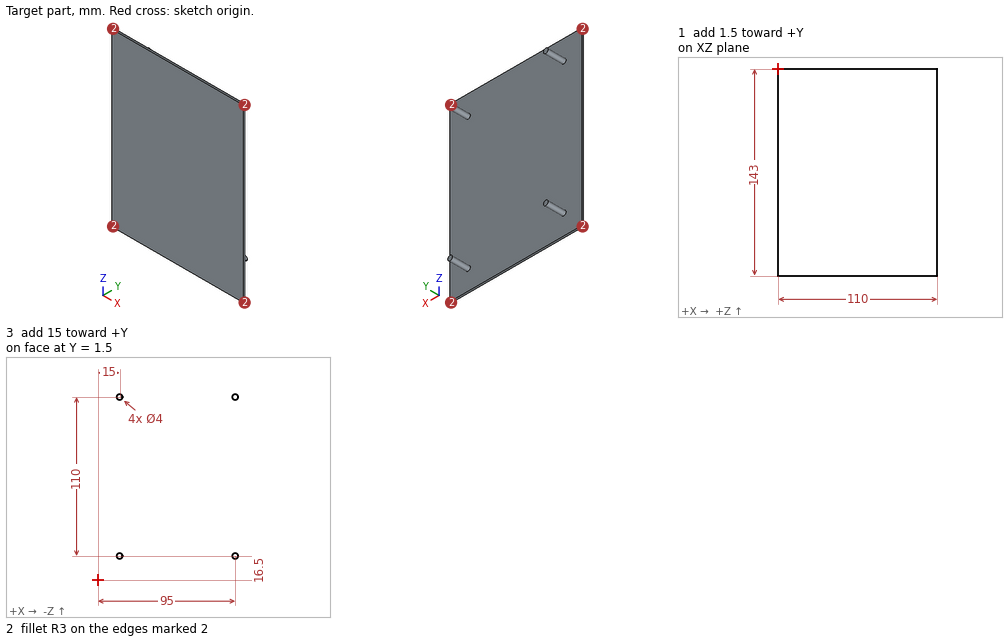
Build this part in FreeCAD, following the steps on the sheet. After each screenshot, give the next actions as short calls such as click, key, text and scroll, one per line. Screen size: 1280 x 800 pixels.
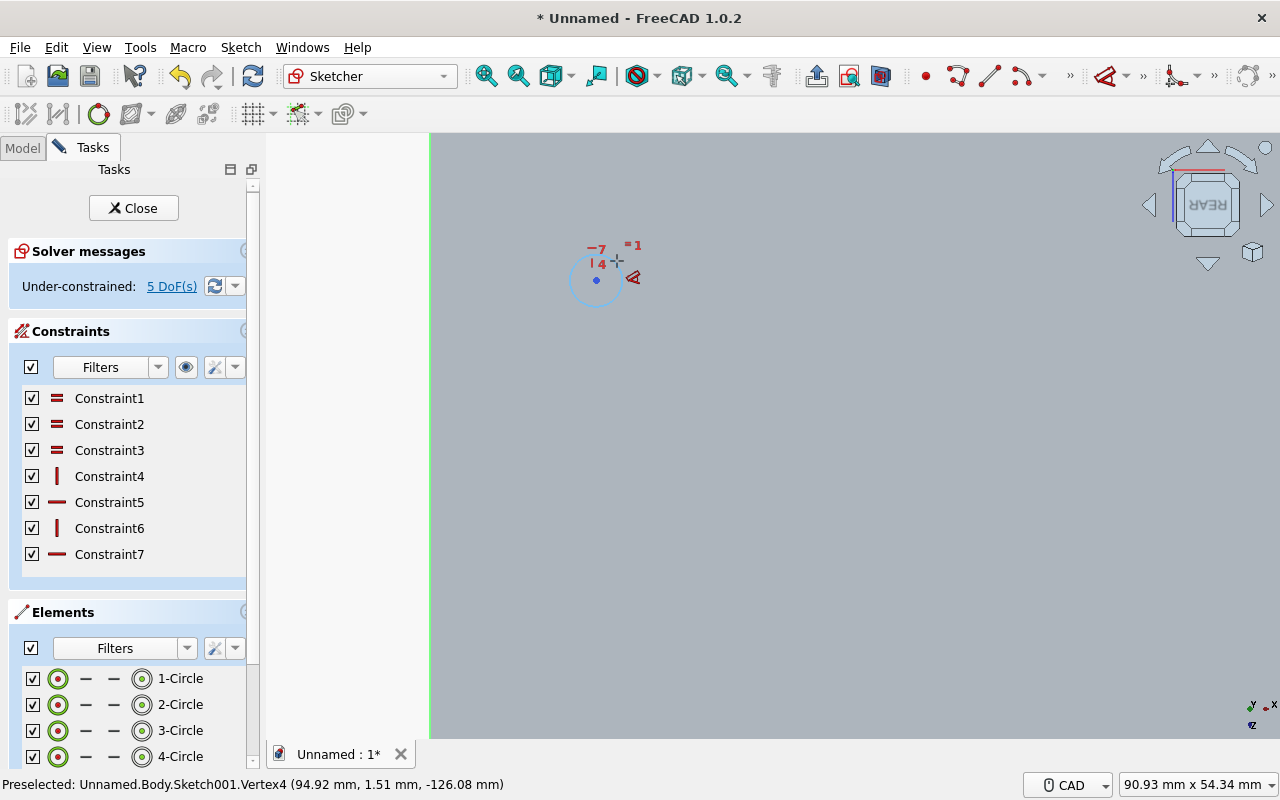
click(614, 262)
click(636, 239)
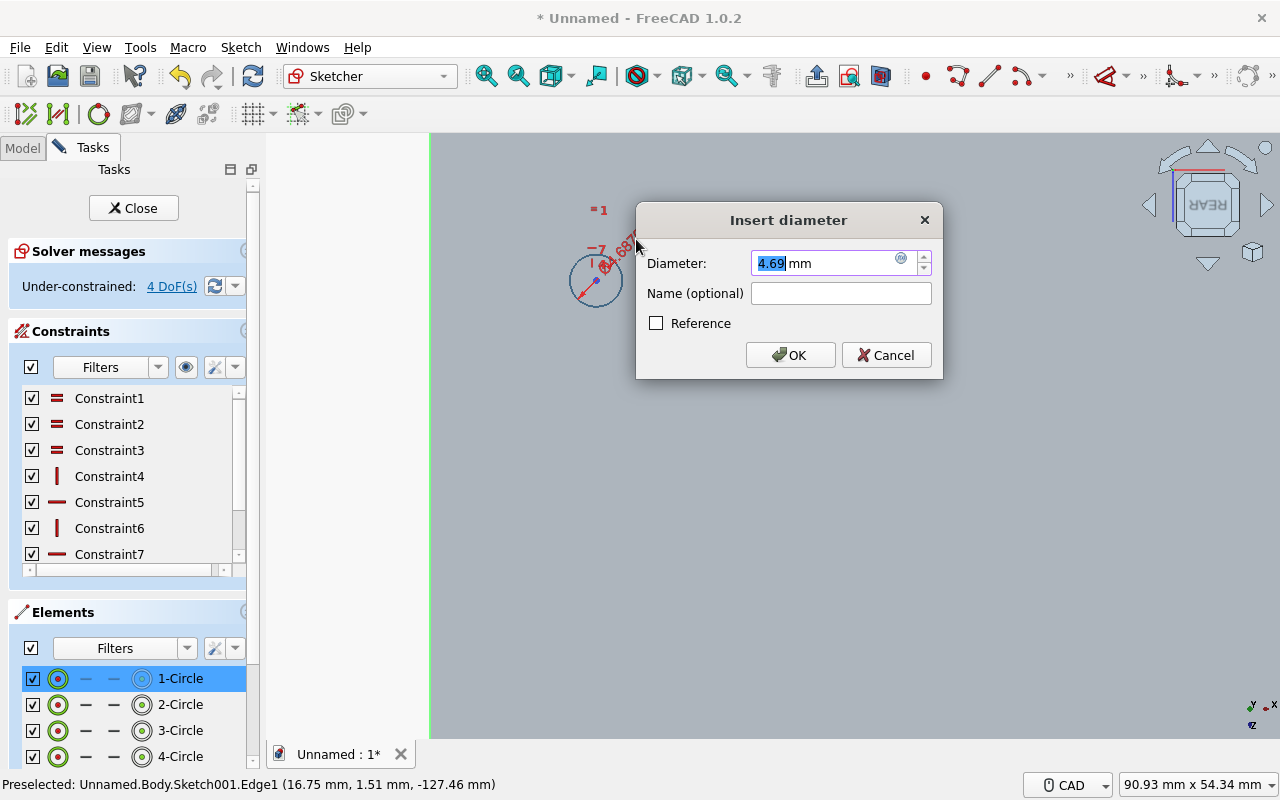
text(4)
key(Return)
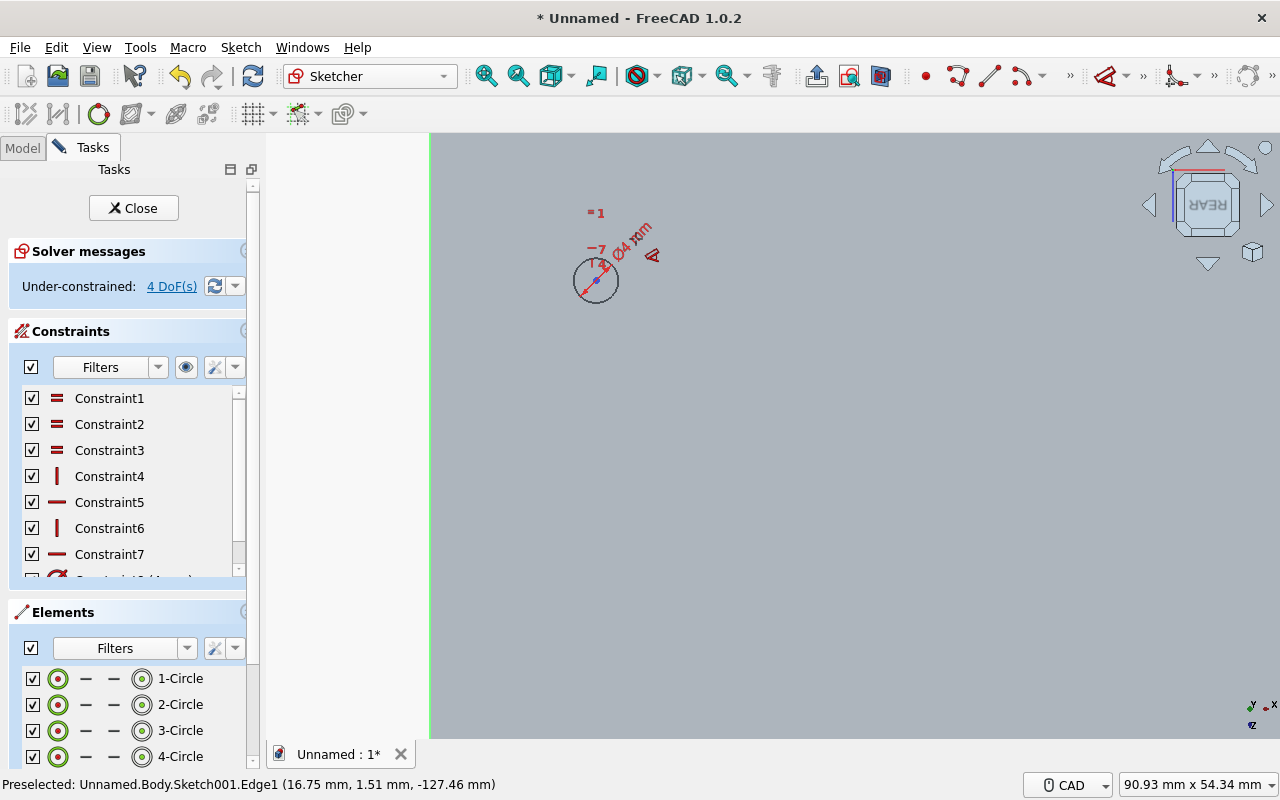
click(596, 281)
click(513, 247)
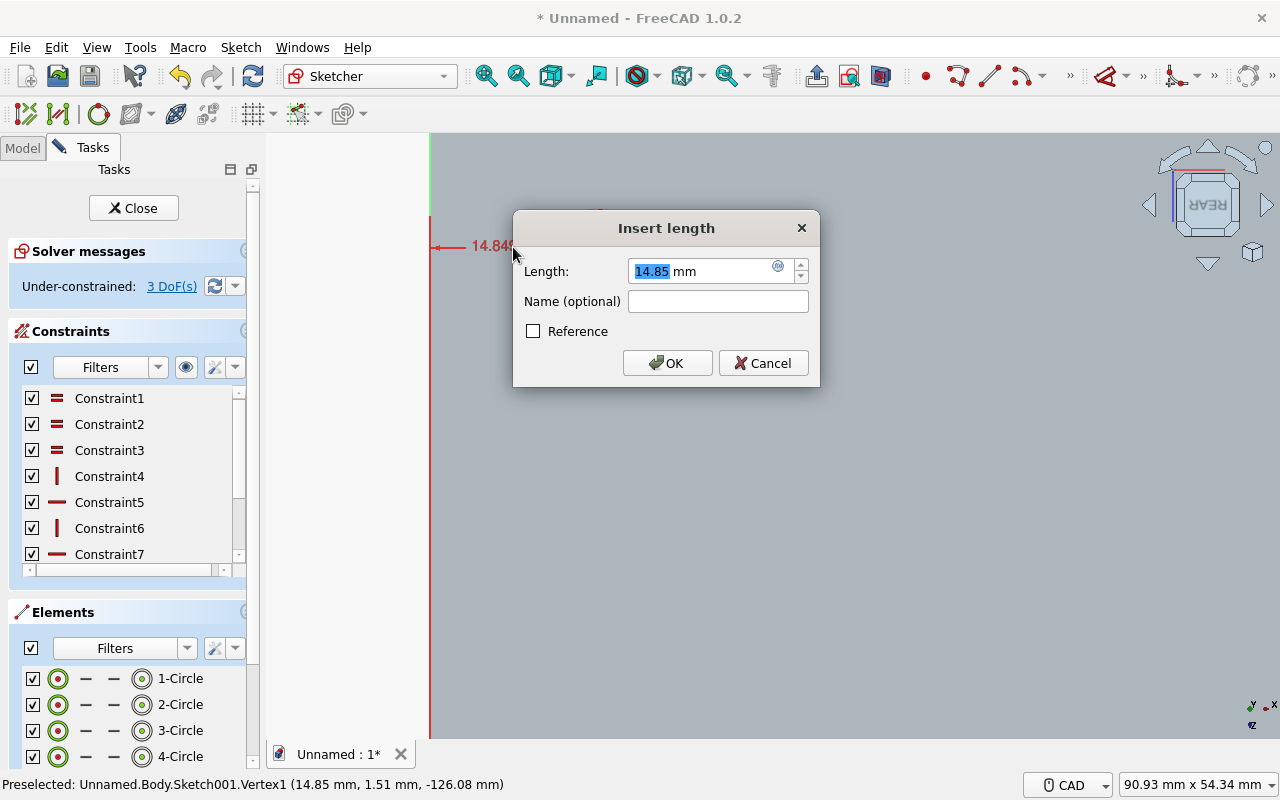
text(15)
key(Return)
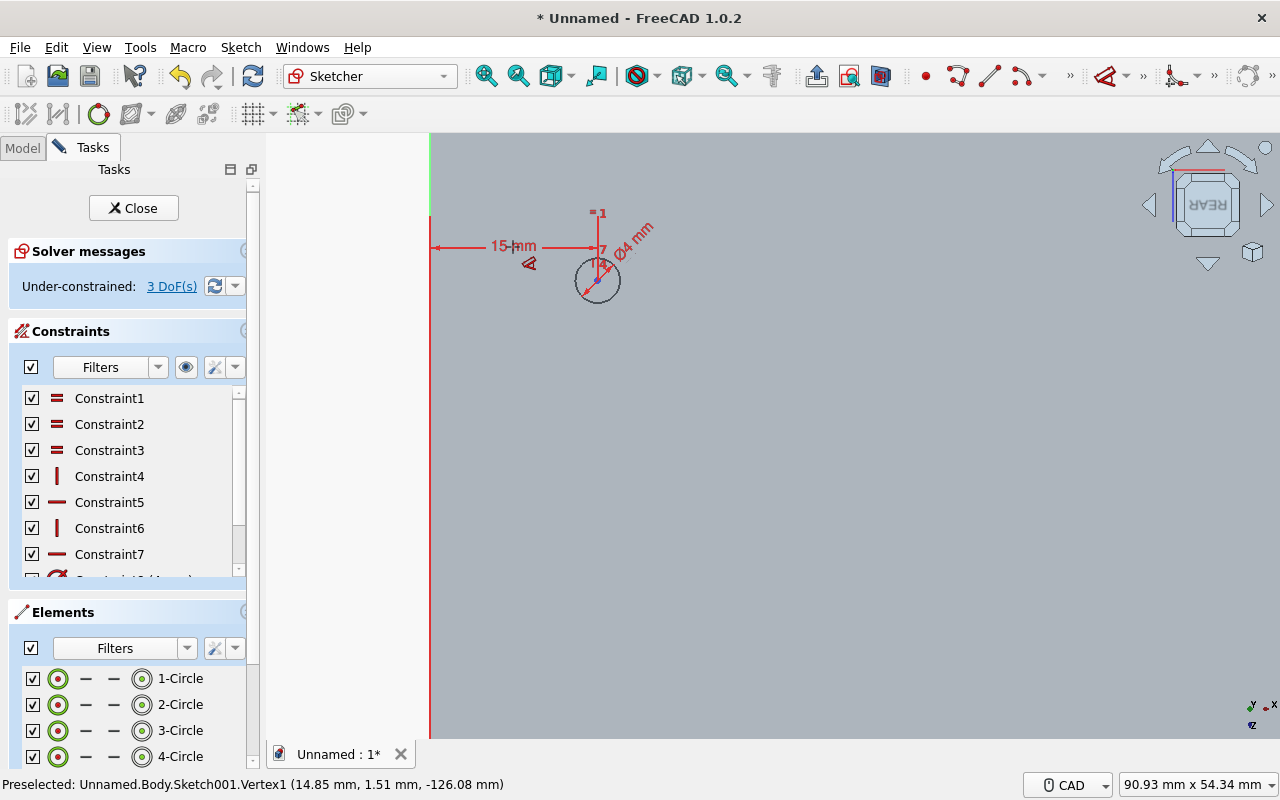
scroll(617, 261, down, 7)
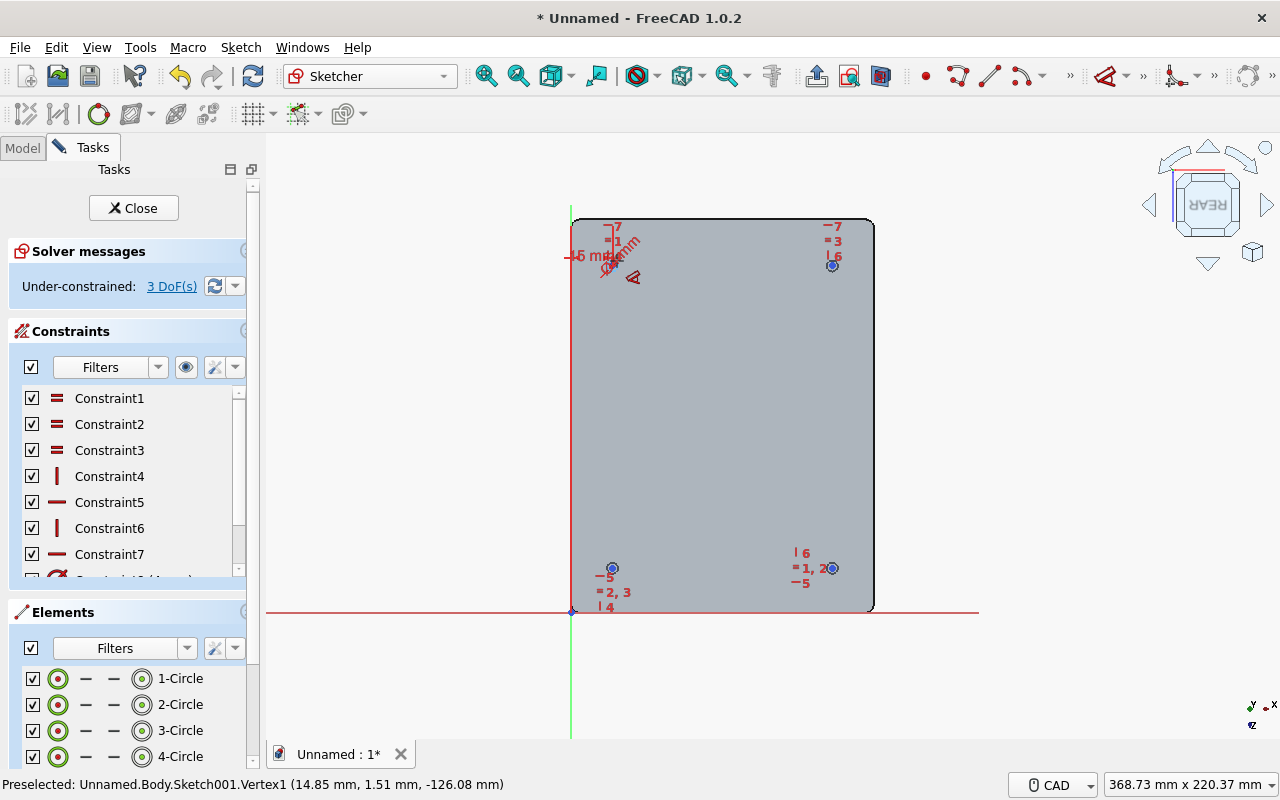
click(832, 568)
click(702, 647)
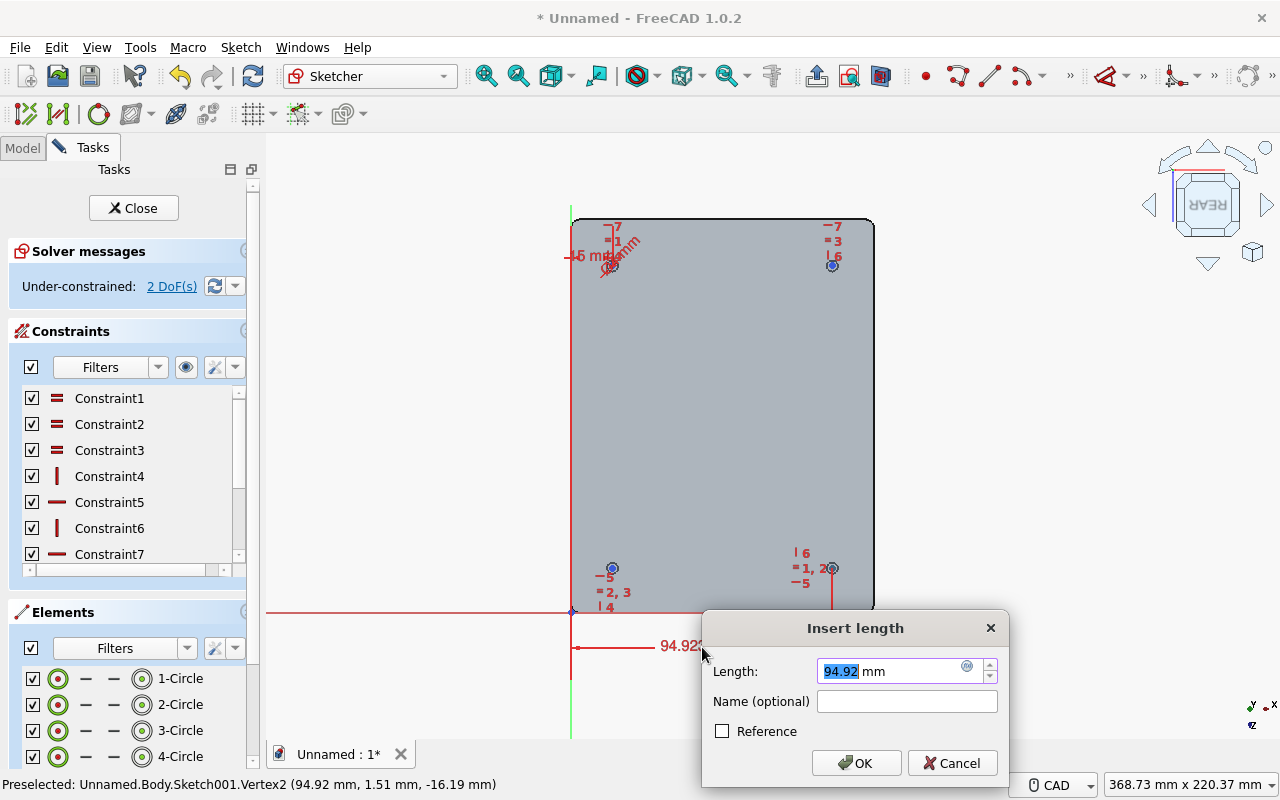
text(95)
key(Return)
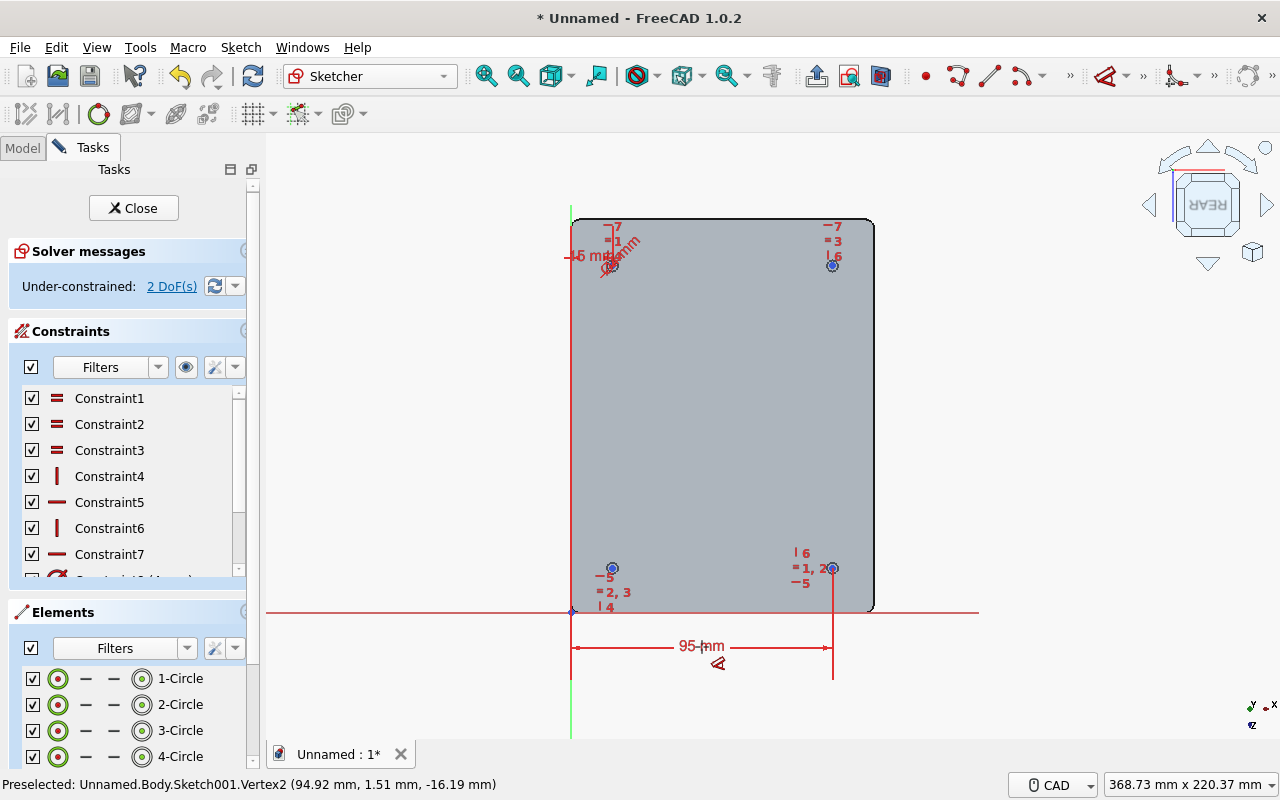
click(833, 568)
click(537, 590)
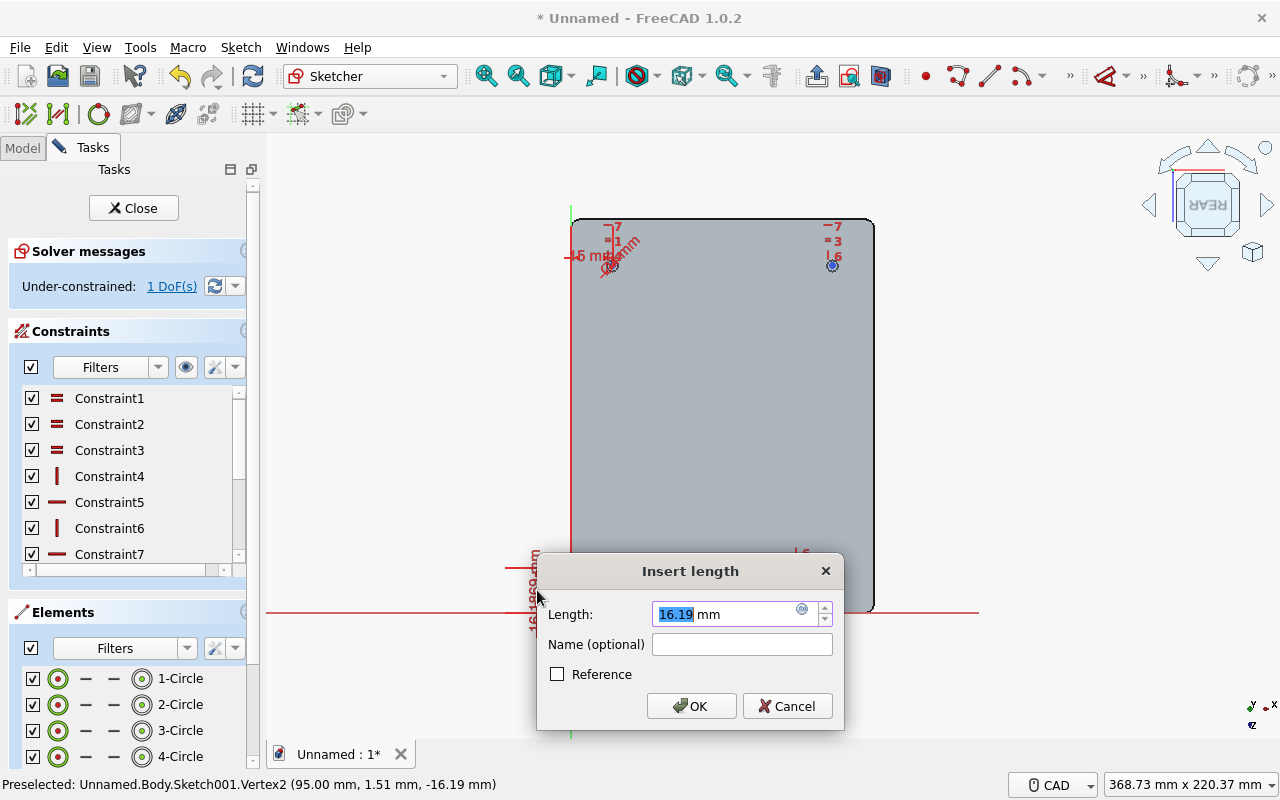
text(16.5)
key(Return)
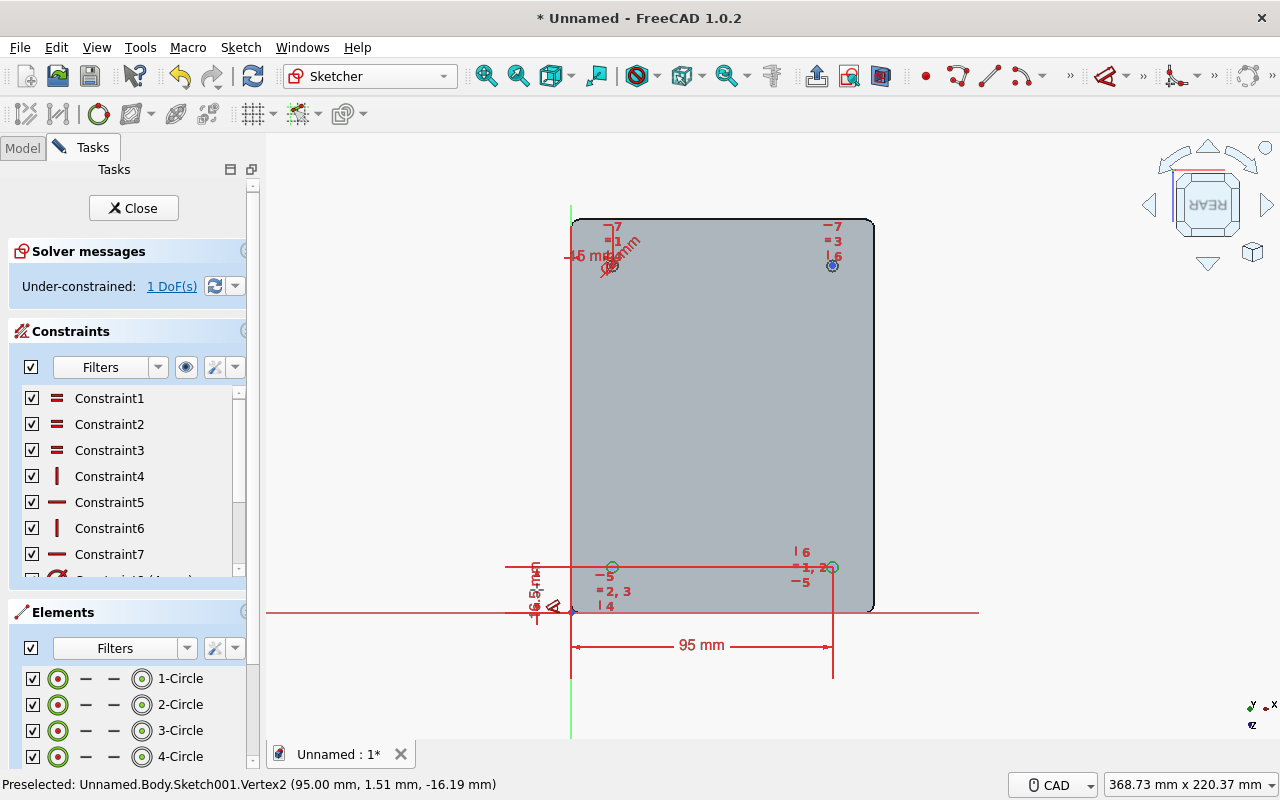
click(613, 266)